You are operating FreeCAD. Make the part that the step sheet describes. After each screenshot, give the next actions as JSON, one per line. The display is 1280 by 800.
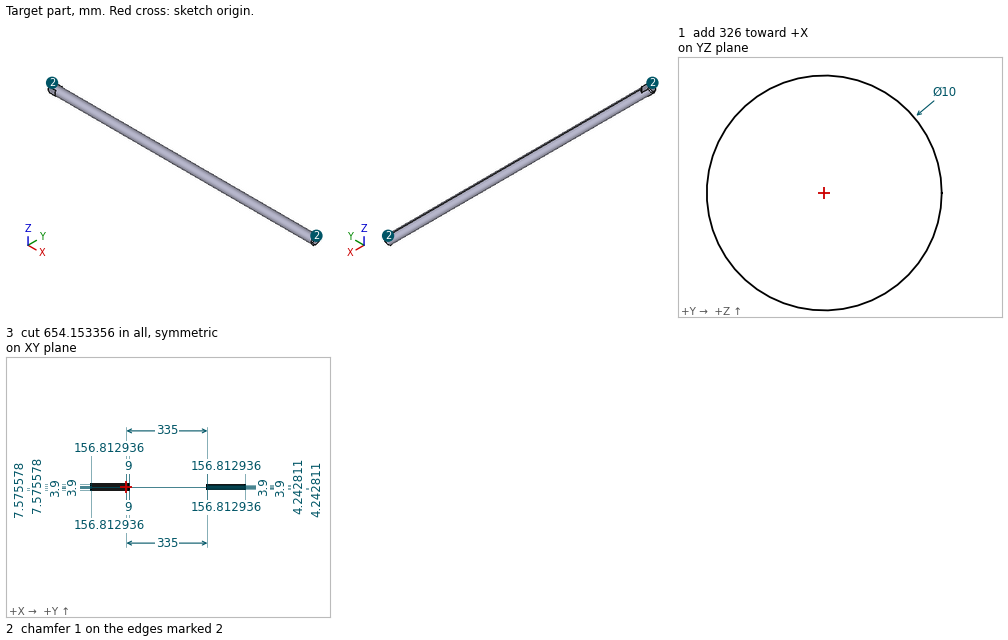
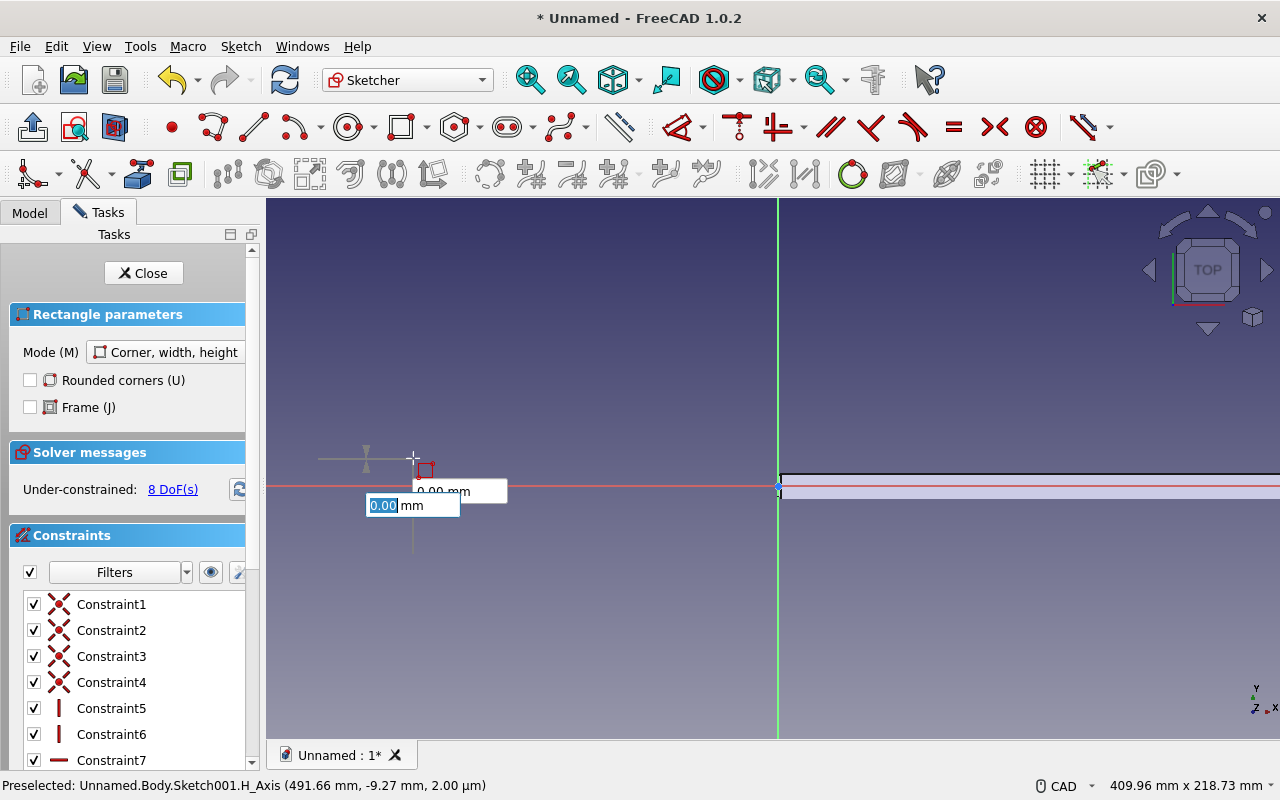
{"action": "scroll", "coordinate": [801, 477], "scroll_direction": "up", "scroll_amount": 3}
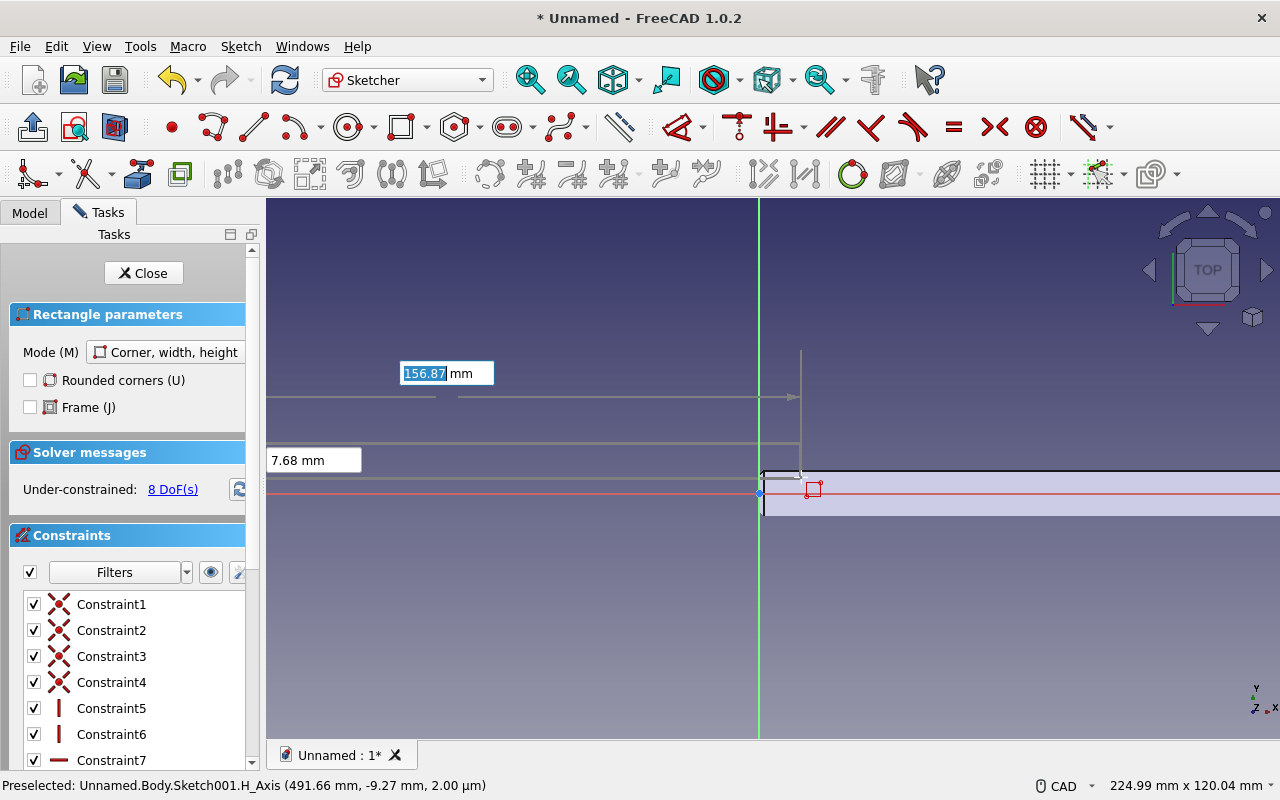
{"action": "left_click", "coordinate": [800, 476]}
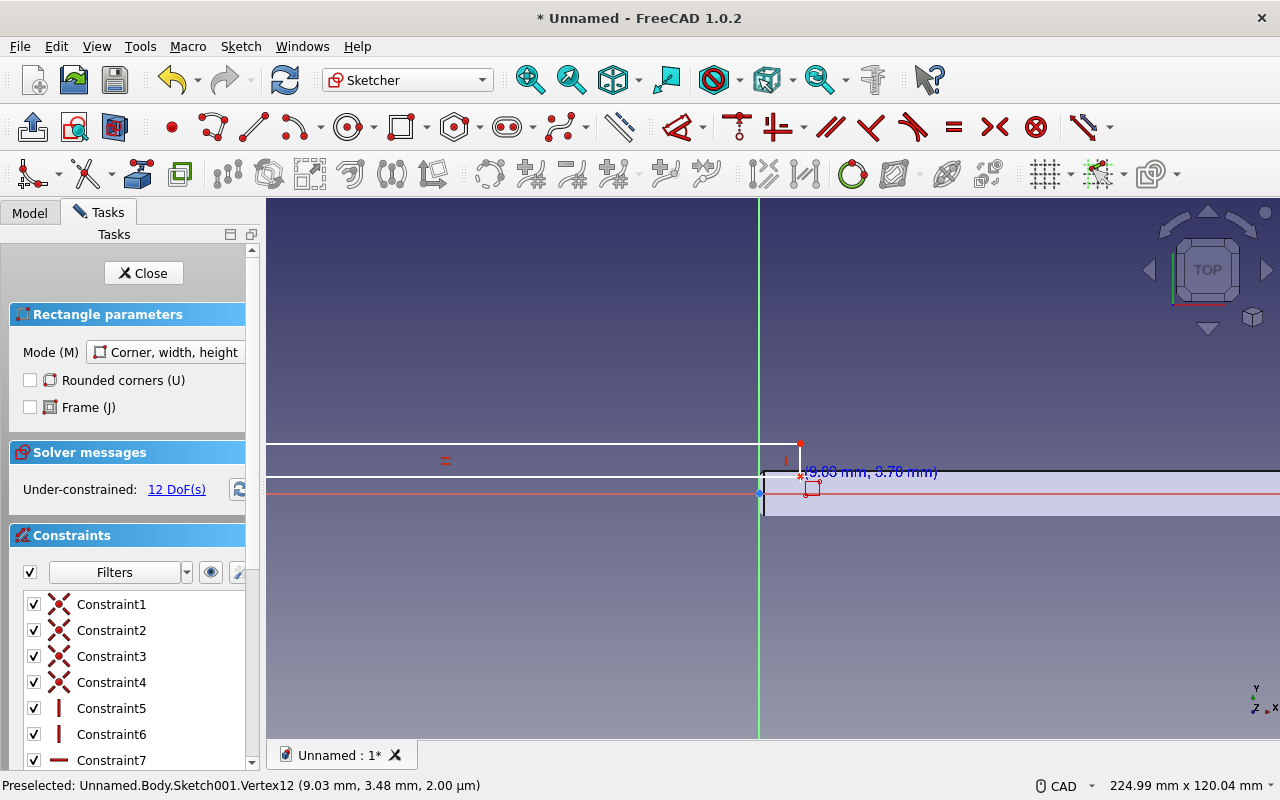
{"action": "scroll", "coordinate": [495, 462], "scroll_direction": "down", "scroll_amount": 8}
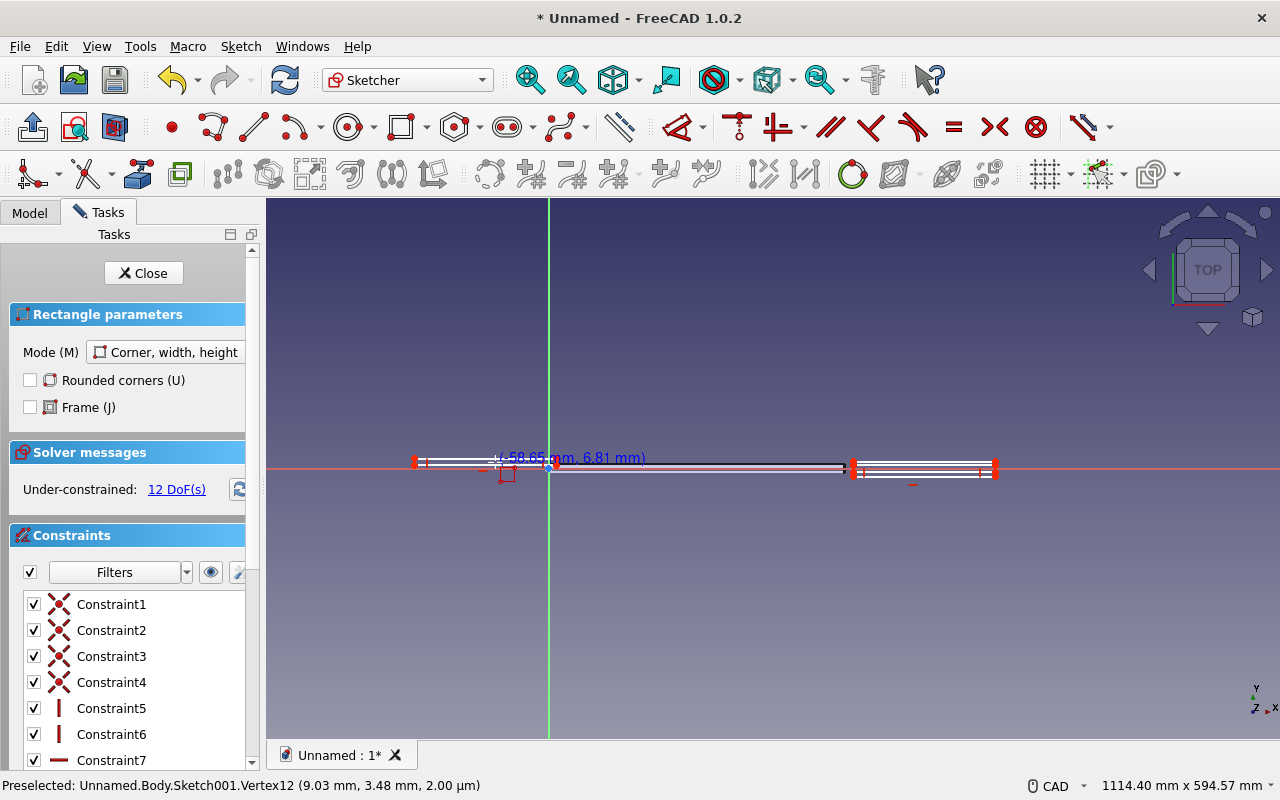
{"action": "scroll", "coordinate": [414, 472], "scroll_direction": "up", "scroll_amount": 8}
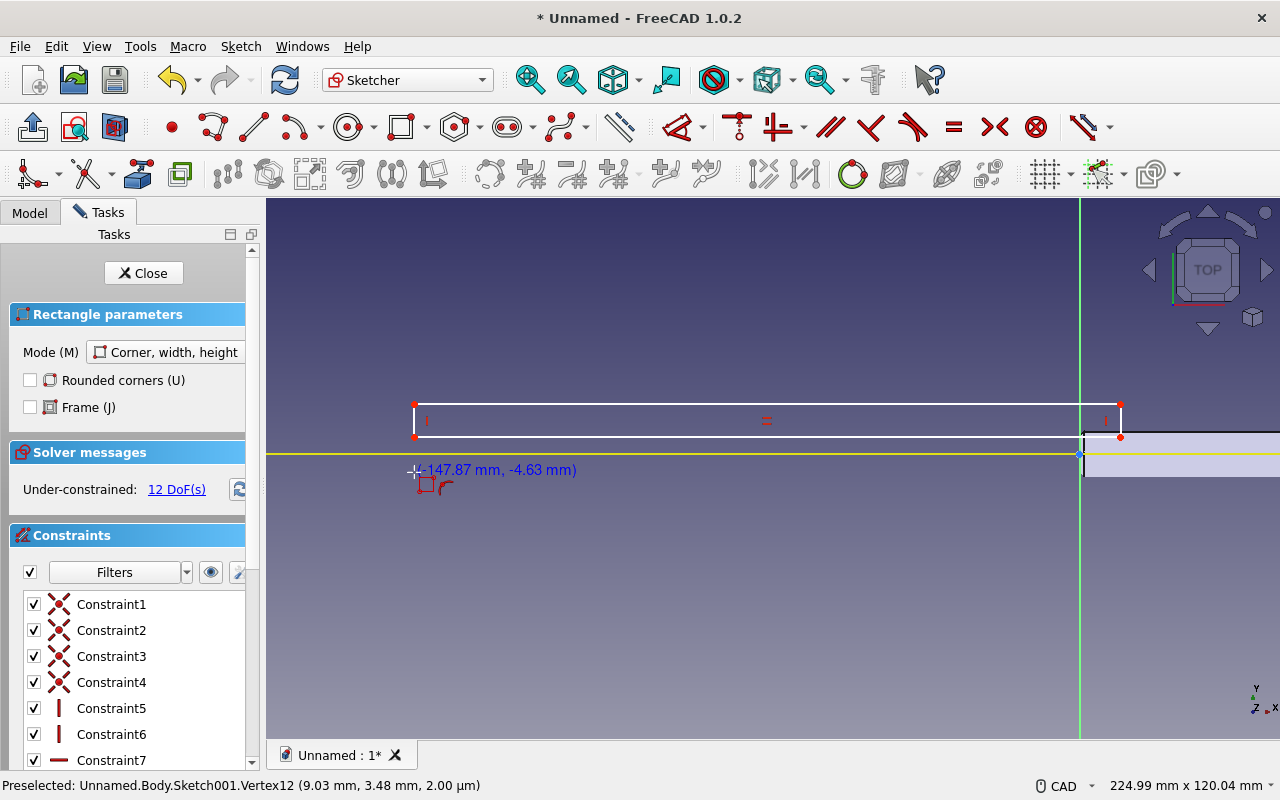
{"action": "left_click", "coordinate": [414, 472]}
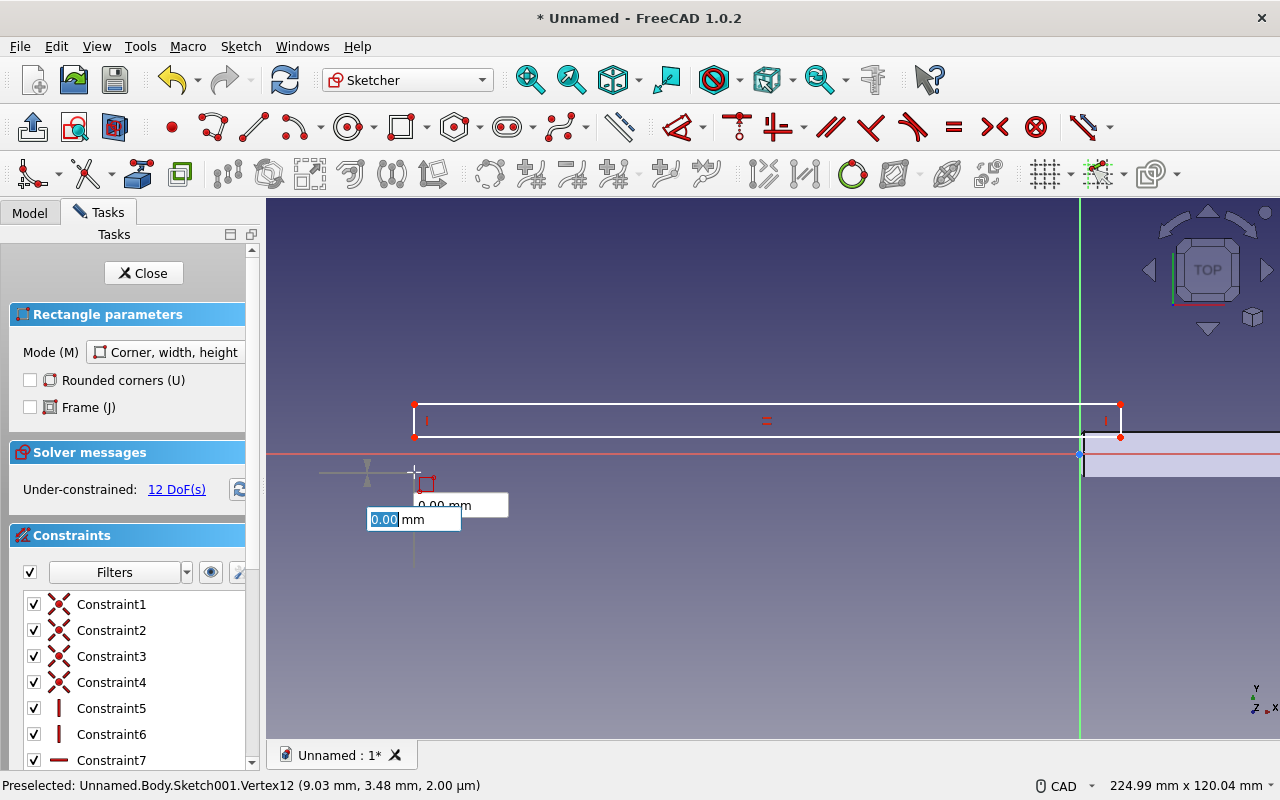
{"action": "scroll", "coordinate": [413, 472], "scroll_direction": "down", "scroll_amount": 8}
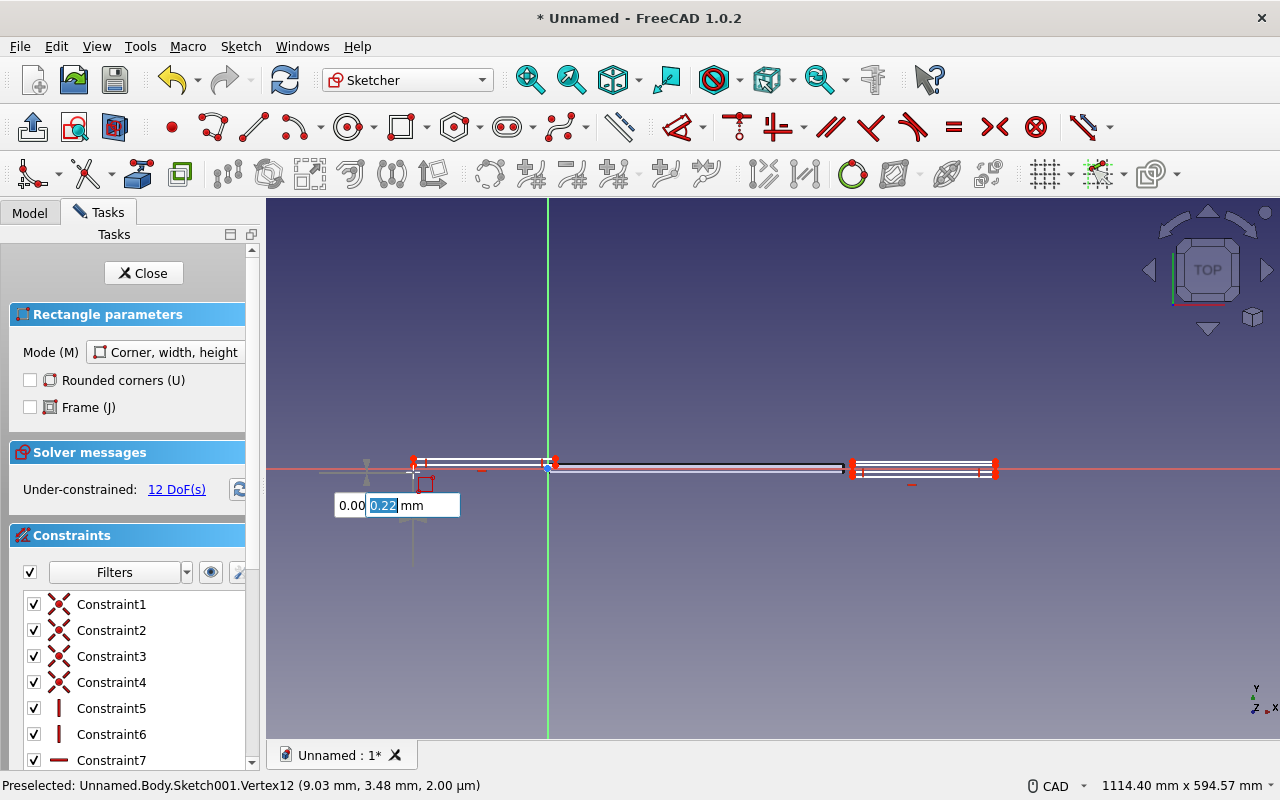
{"action": "scroll", "coordinate": [556, 479], "scroll_direction": "up", "scroll_amount": 4}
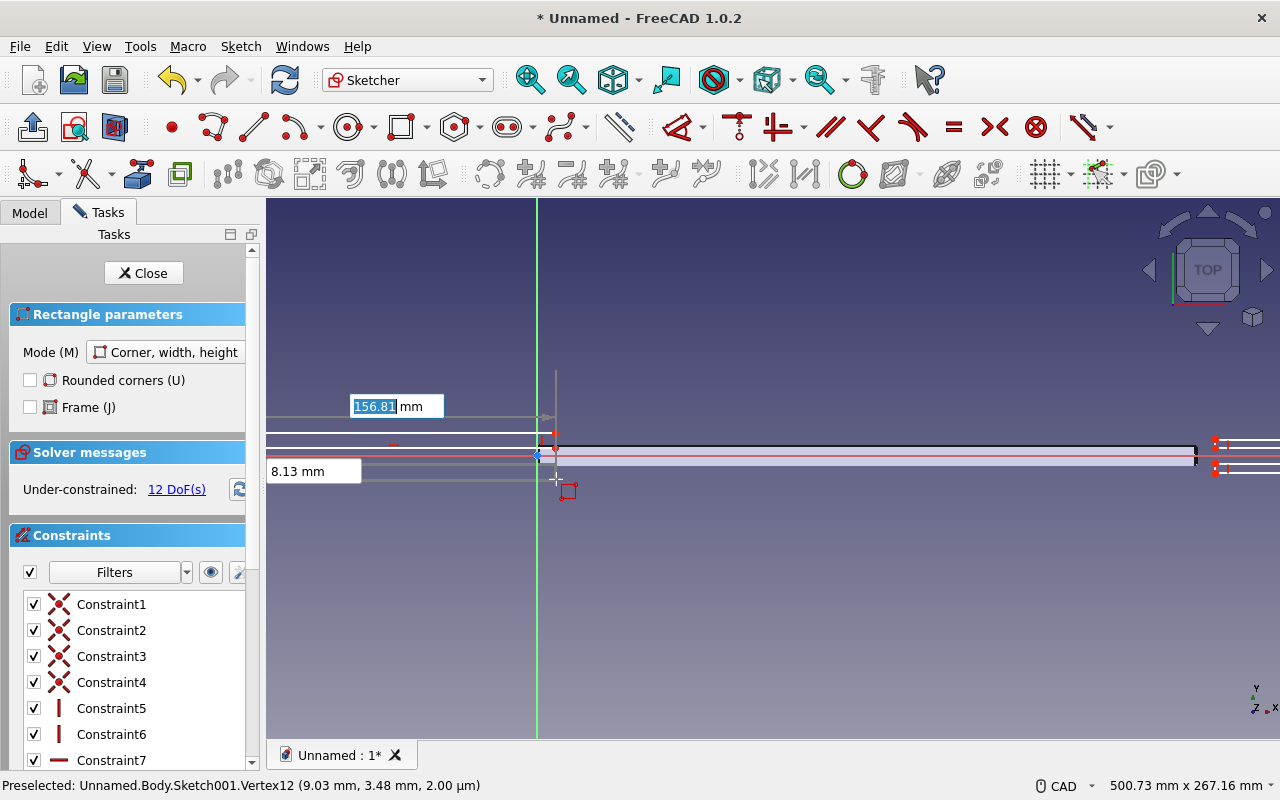
{"action": "left_click", "coordinate": [556, 479]}
{"action": "key", "text": "Escape"}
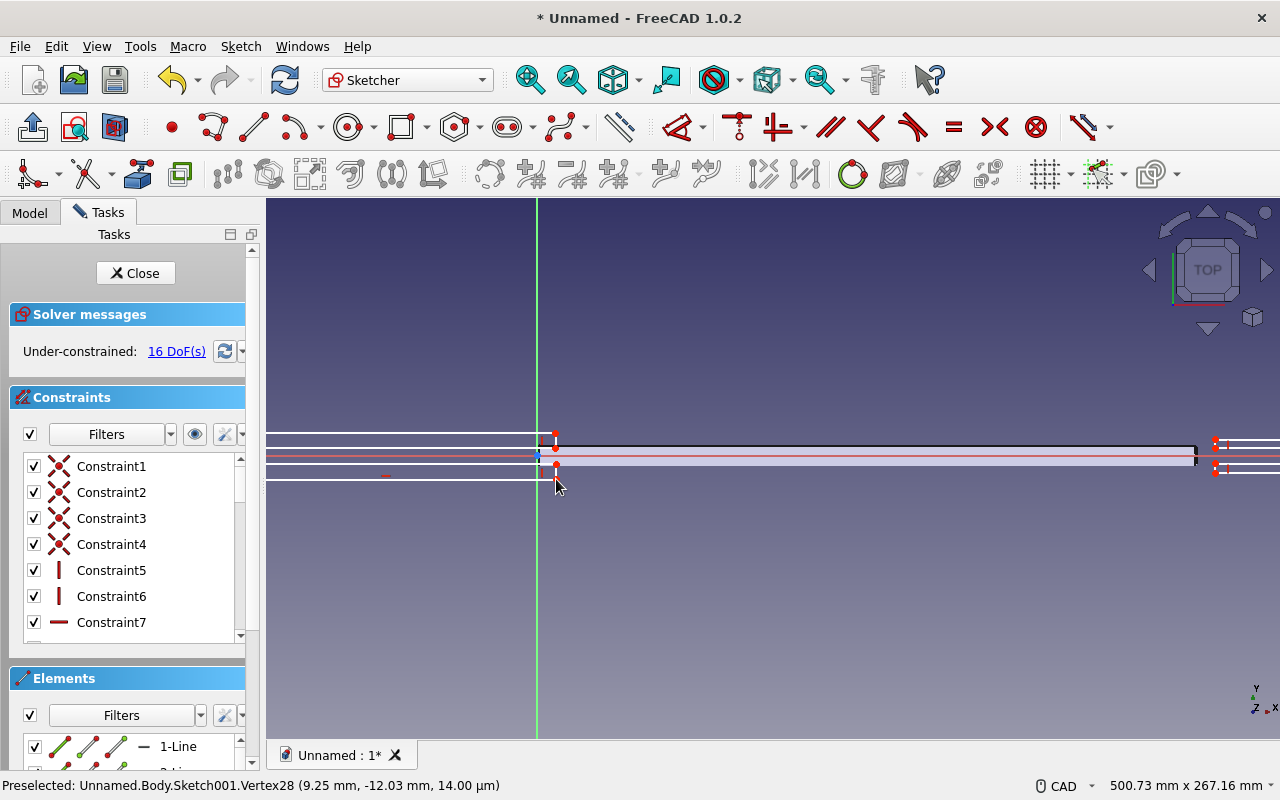
{"action": "left_click", "coordinate": [676, 128]}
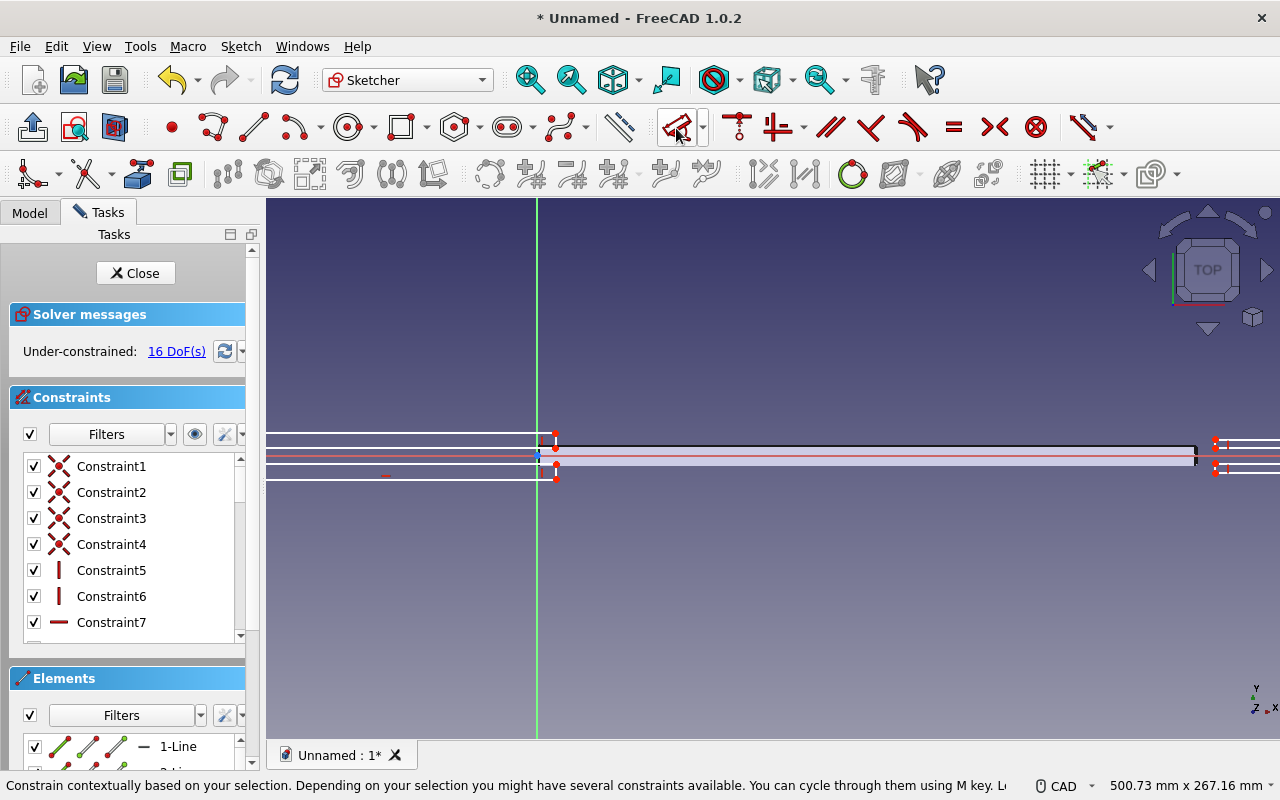
{"action": "scroll", "coordinate": [556, 448], "scroll_direction": "up", "scroll_amount": 4}